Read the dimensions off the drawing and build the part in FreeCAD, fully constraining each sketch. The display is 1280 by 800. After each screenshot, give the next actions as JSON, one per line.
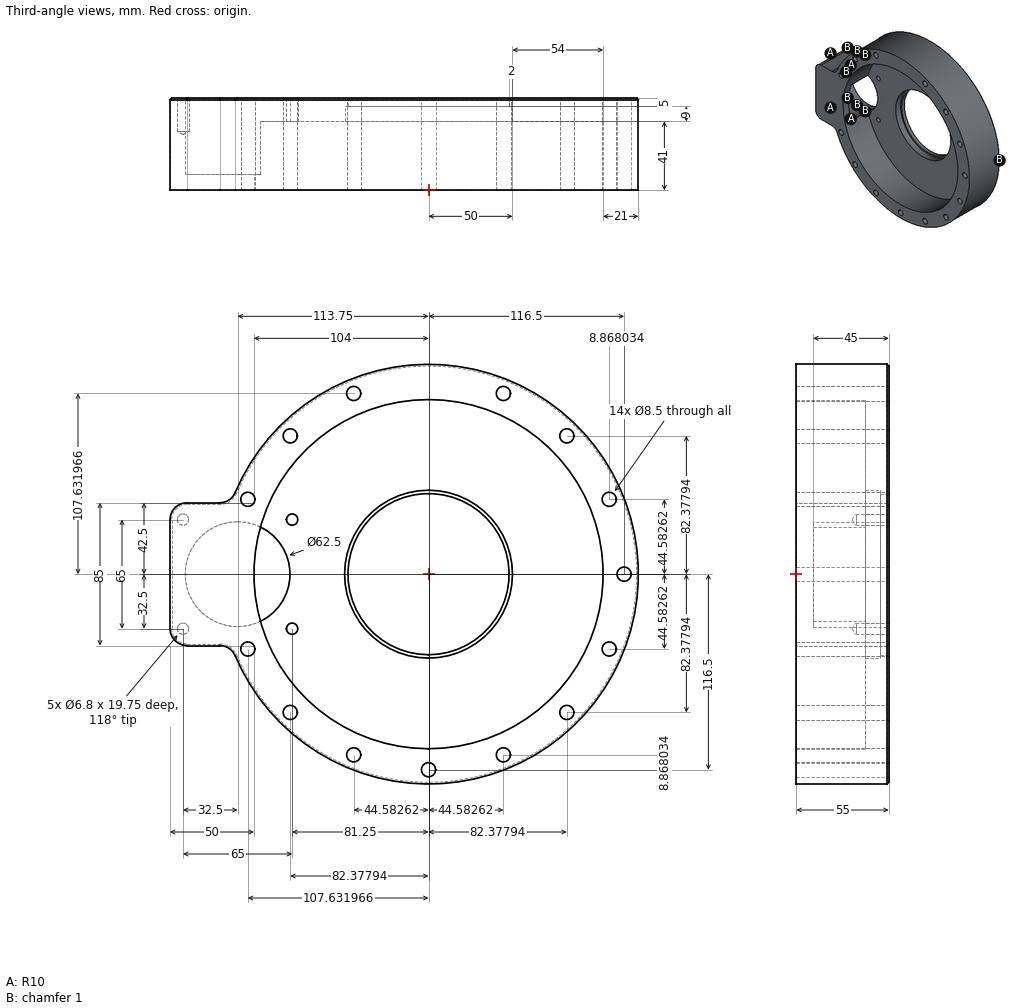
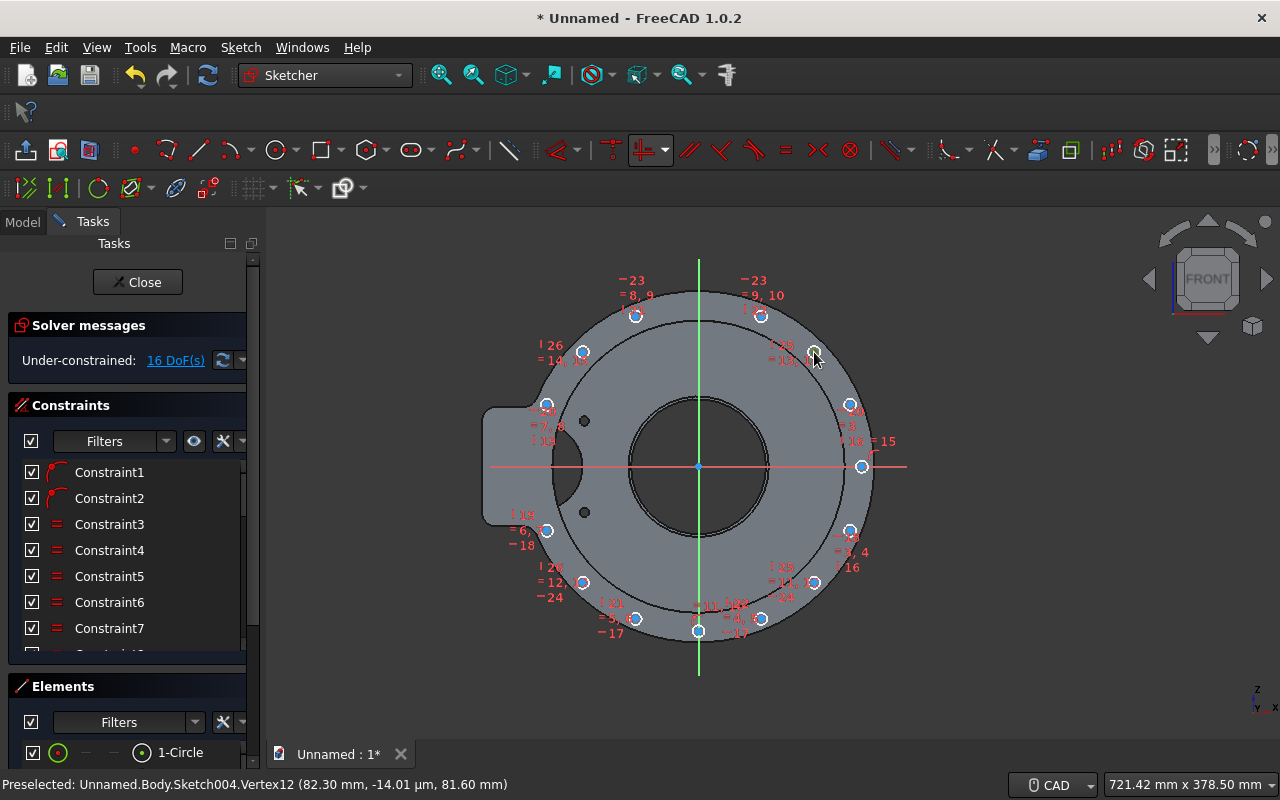
{"action": "scroll", "coordinate": [583, 352], "scroll_direction": "up", "scroll_amount": 4}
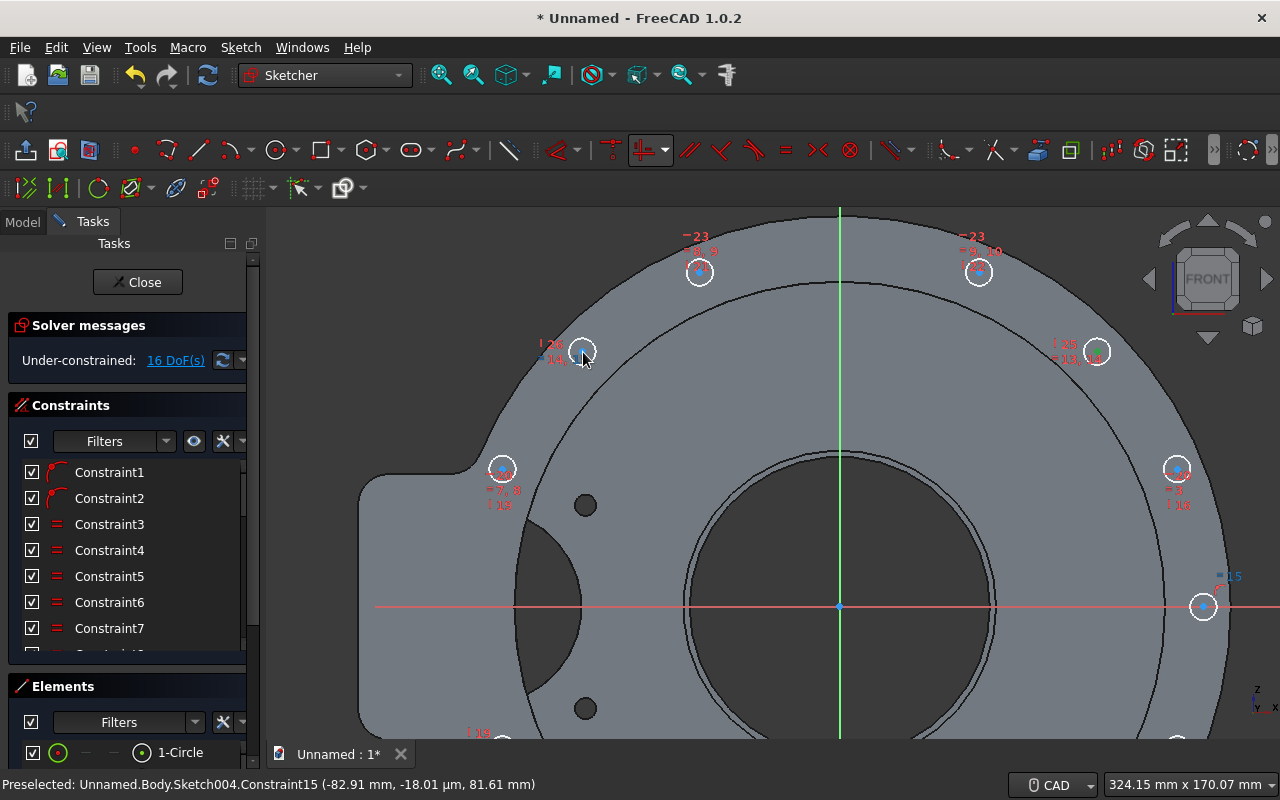
{"action": "scroll", "coordinate": [582, 352], "scroll_direction": "up", "scroll_amount": 4}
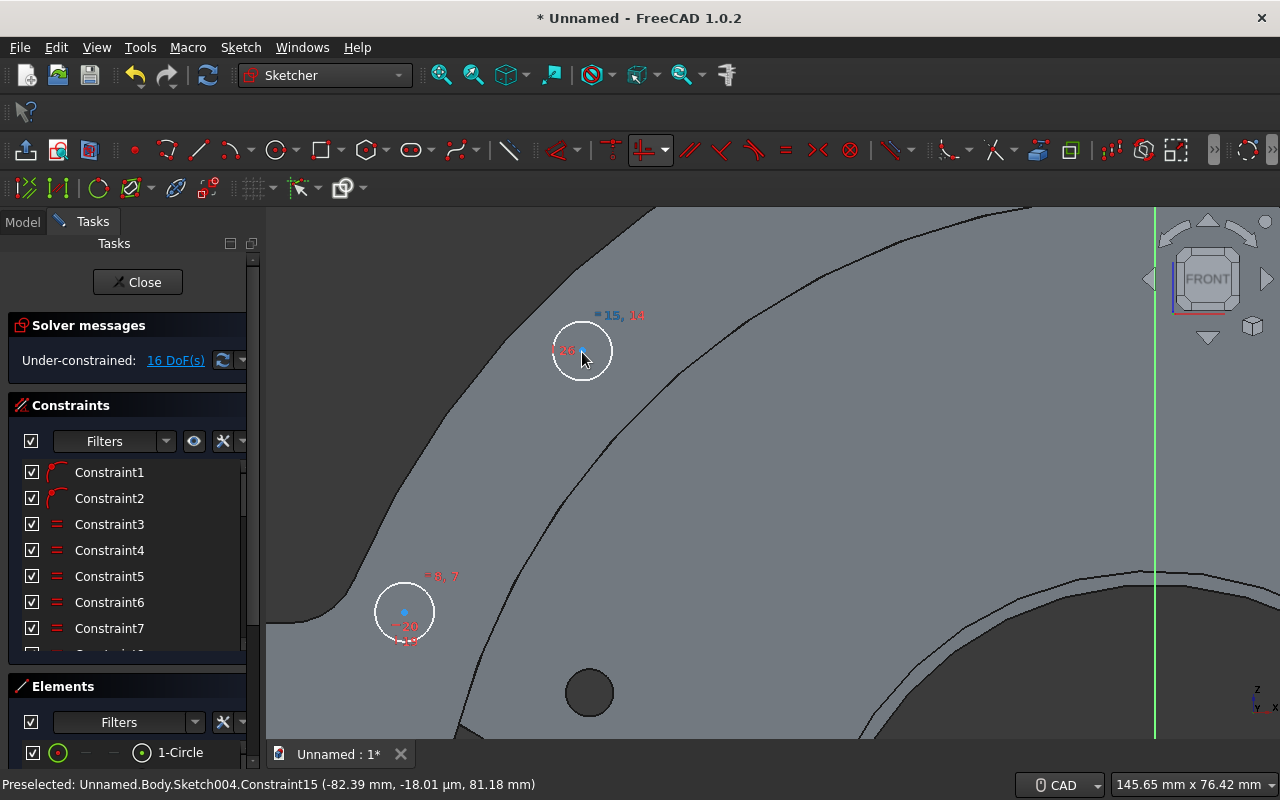
{"action": "left_click", "coordinate": [582, 351]}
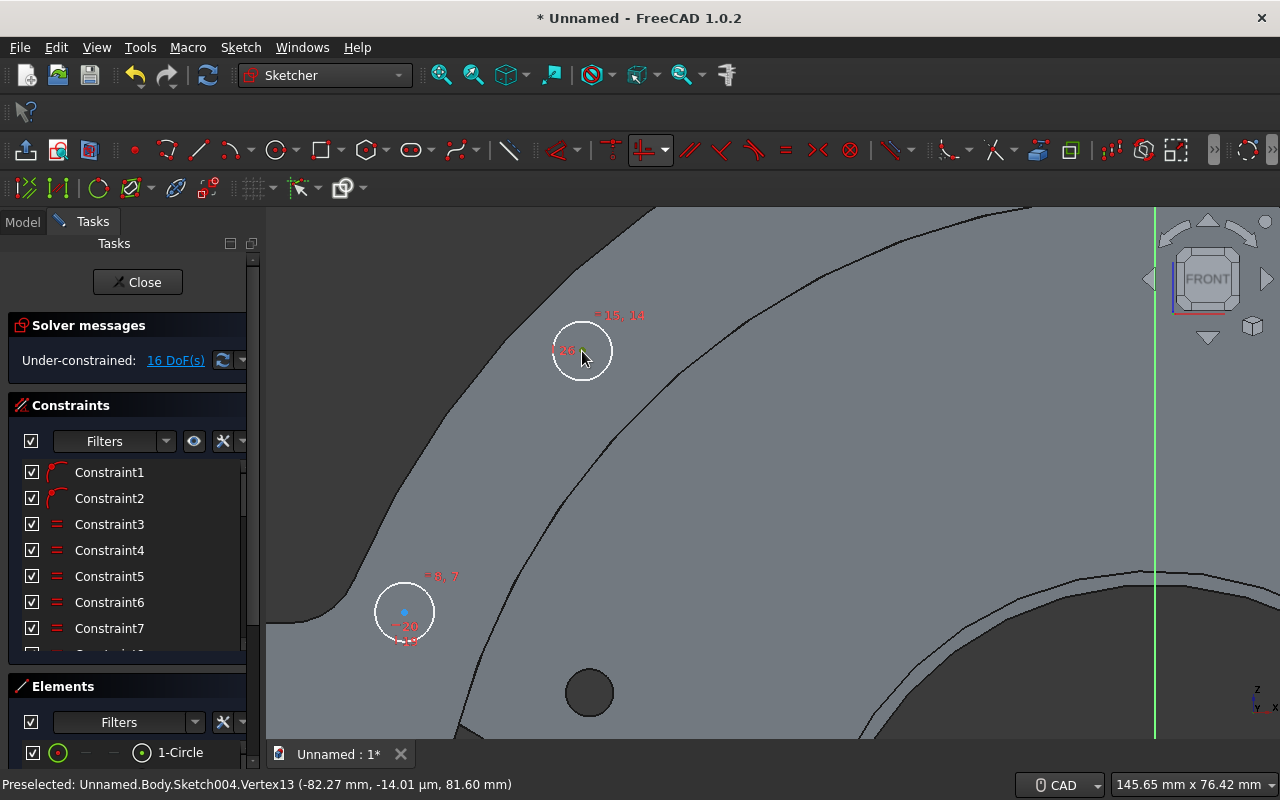
{"action": "key", "text": "h"}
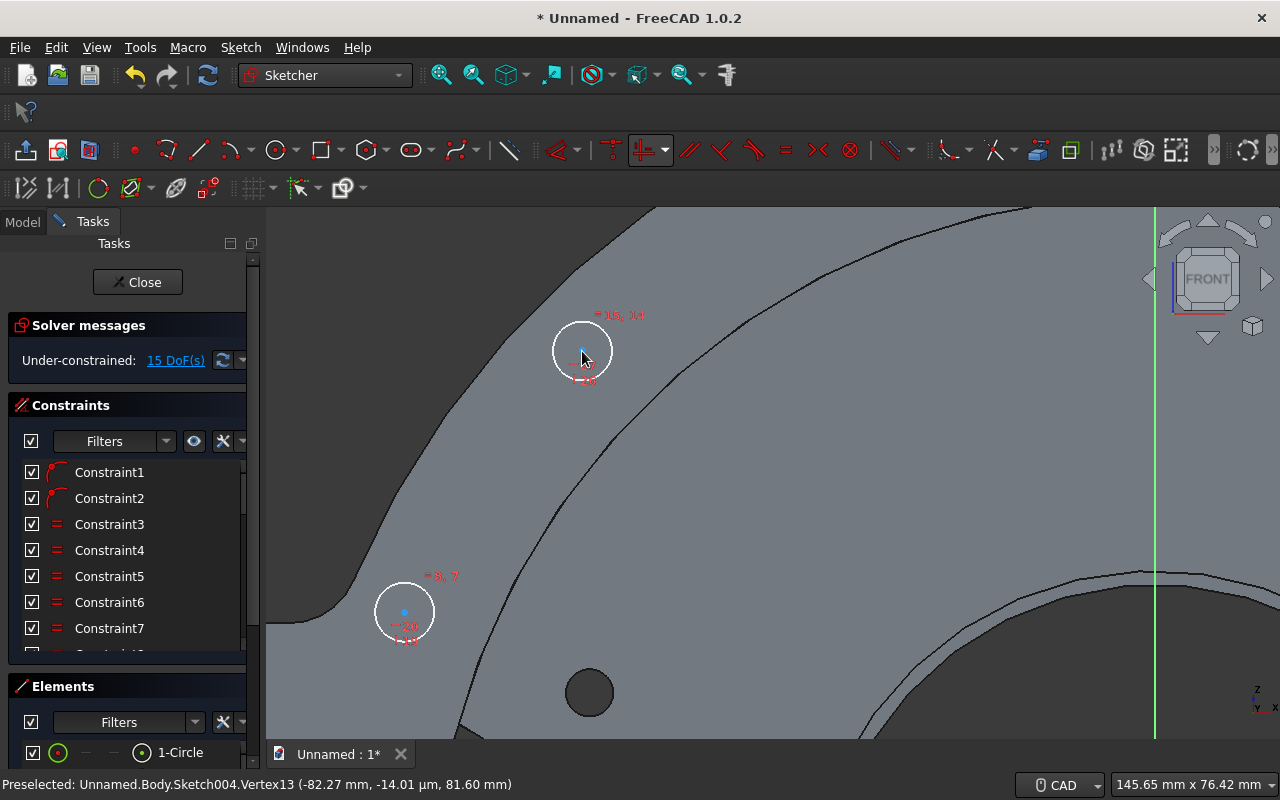
{"action": "key", "text": "d"}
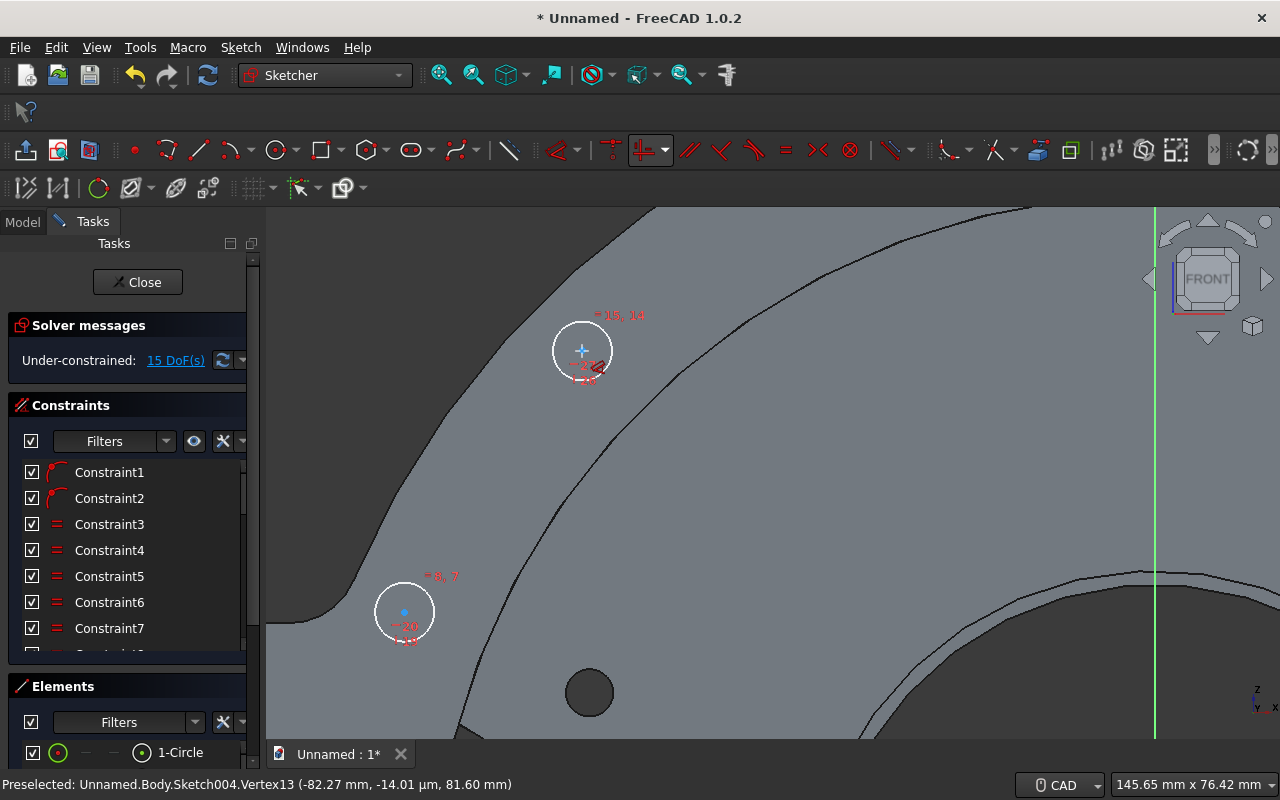
{"action": "scroll", "coordinate": [583, 352], "scroll_direction": "down", "scroll_amount": 8}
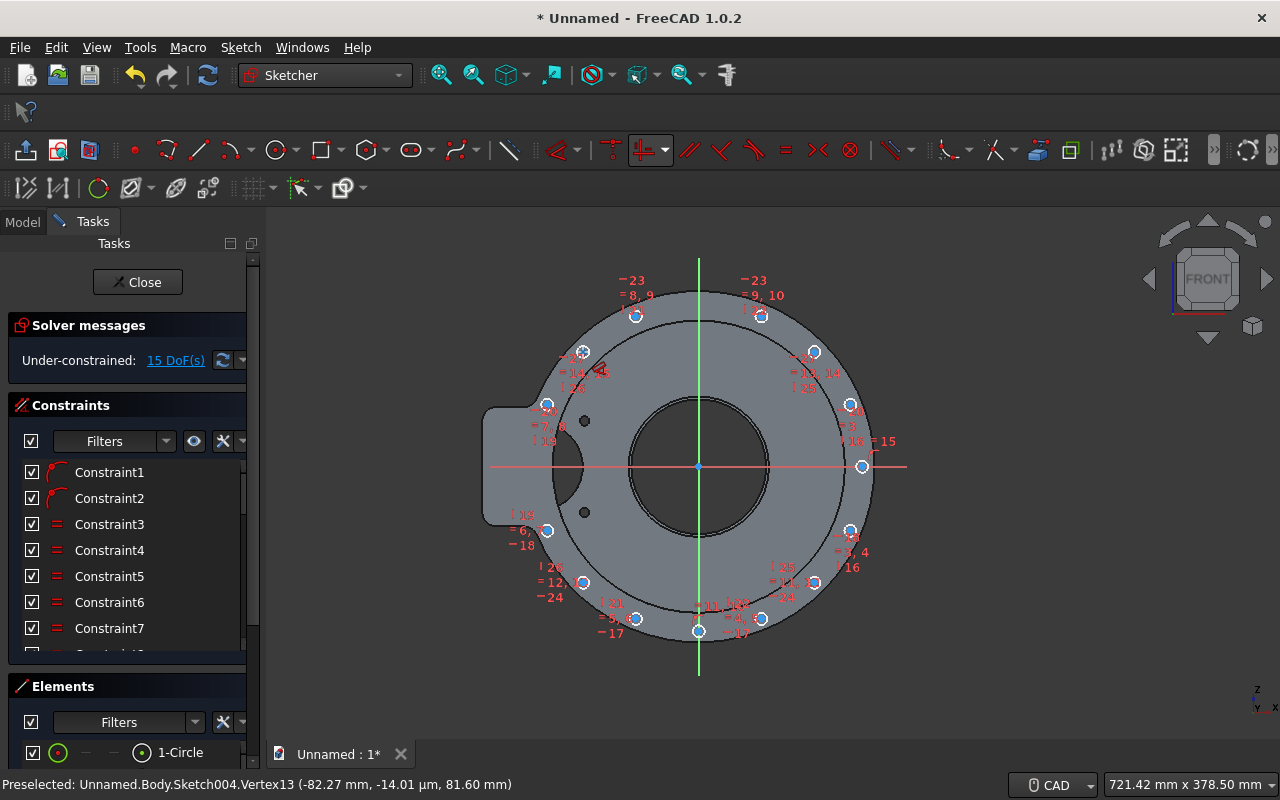
{"action": "scroll", "coordinate": [855, 401], "scroll_direction": "up", "scroll_amount": 7}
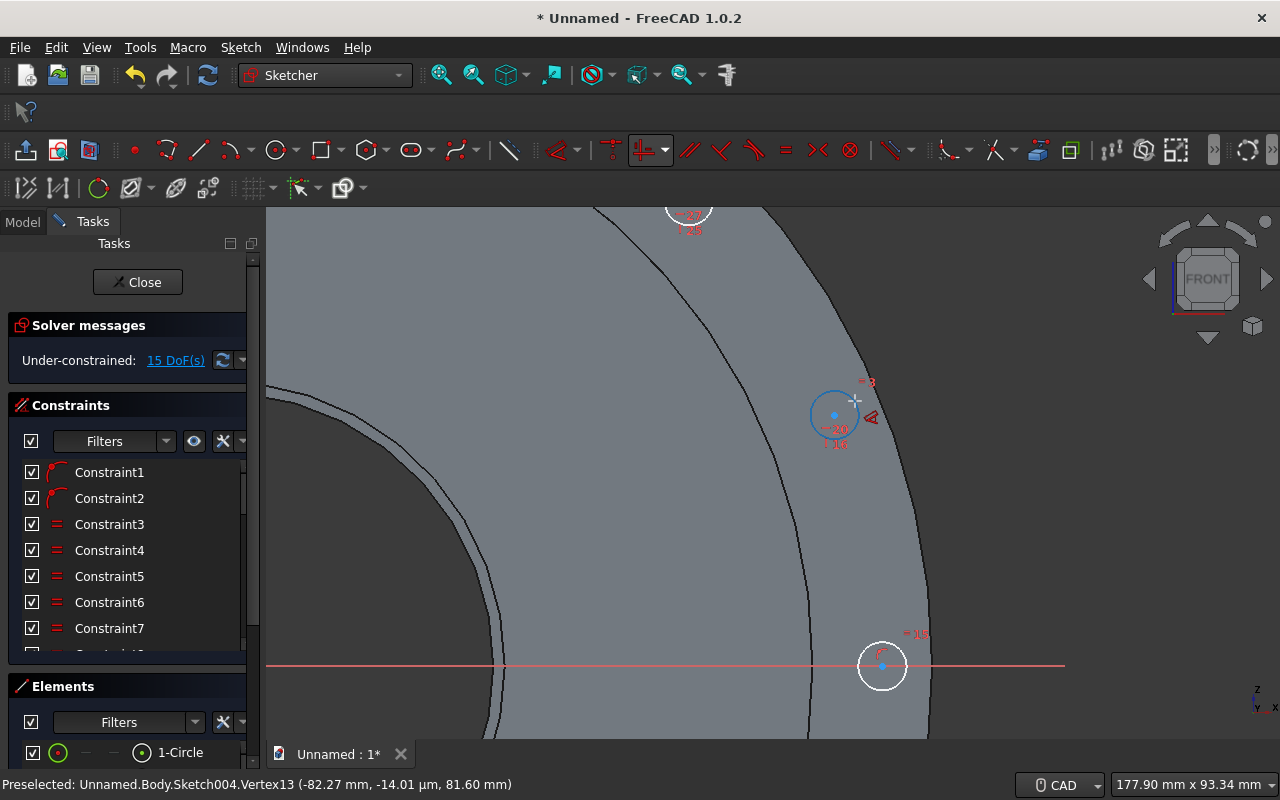
{"action": "left_click", "coordinate": [852, 398]}
{"action": "left_click", "coordinate": [875, 376]}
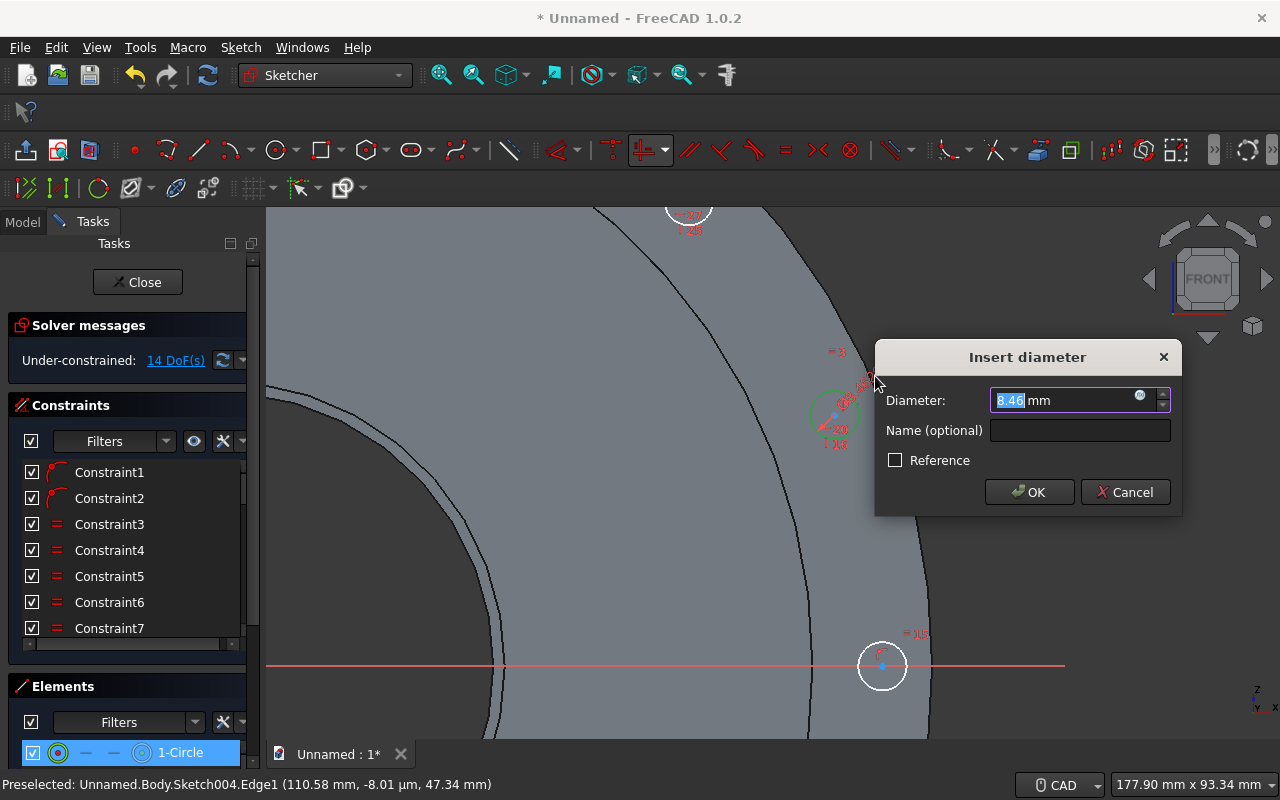
{"action": "type", "text": "8.5"}
{"action": "key", "text": "Return"}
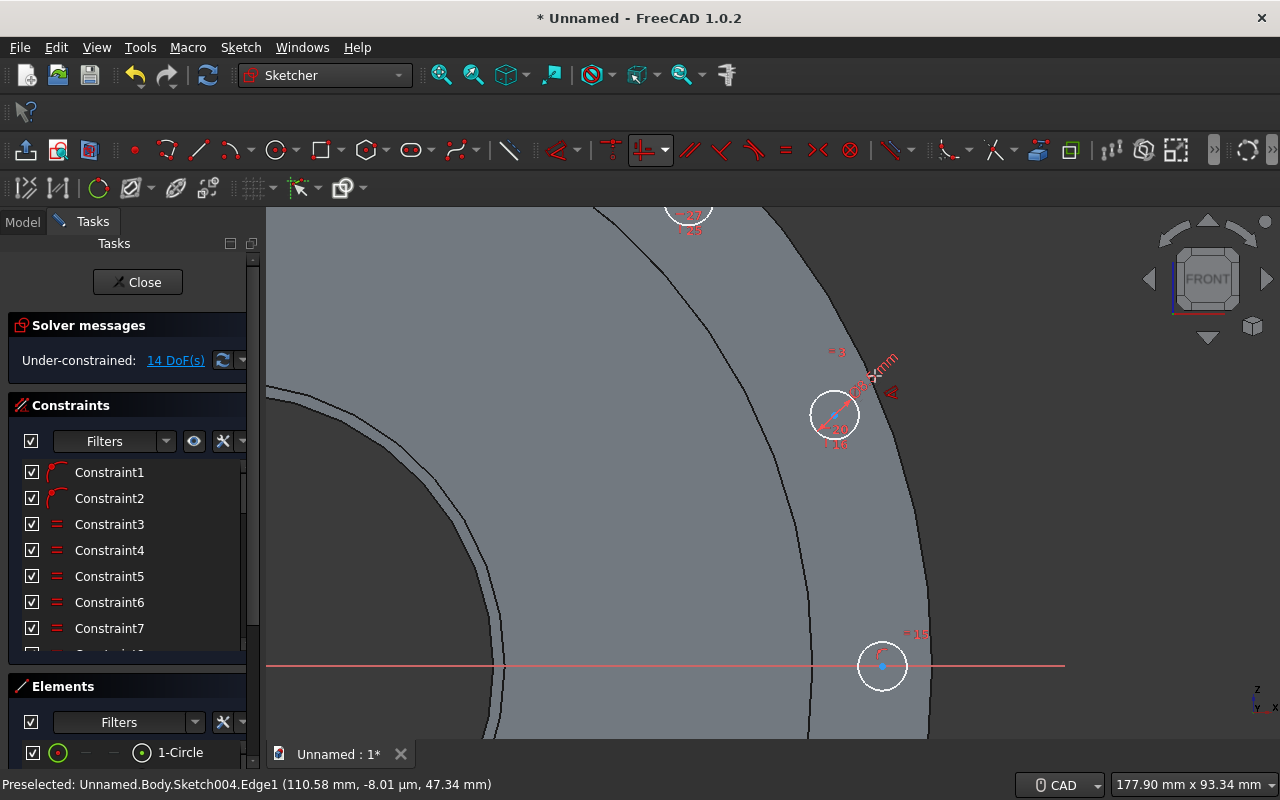
{"action": "scroll", "coordinate": [855, 401], "scroll_direction": "down", "scroll_amount": 7}